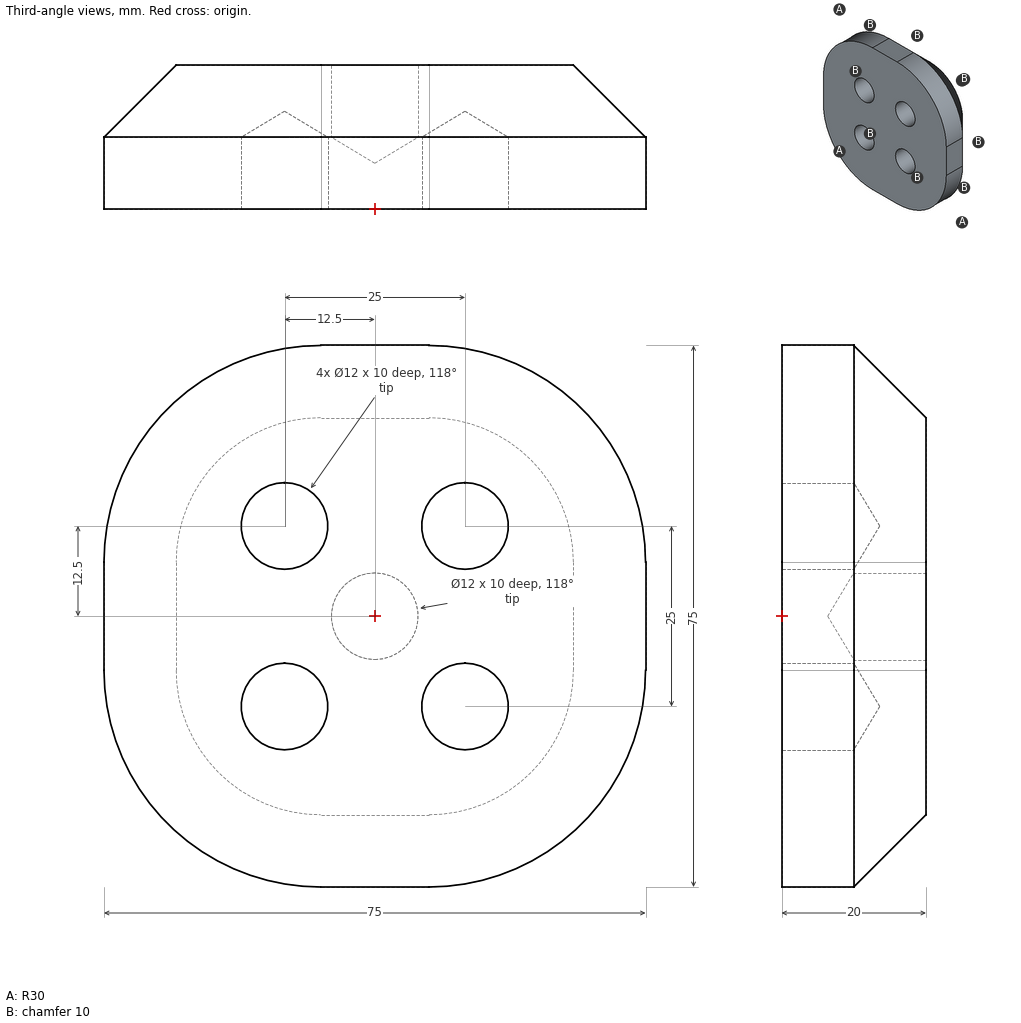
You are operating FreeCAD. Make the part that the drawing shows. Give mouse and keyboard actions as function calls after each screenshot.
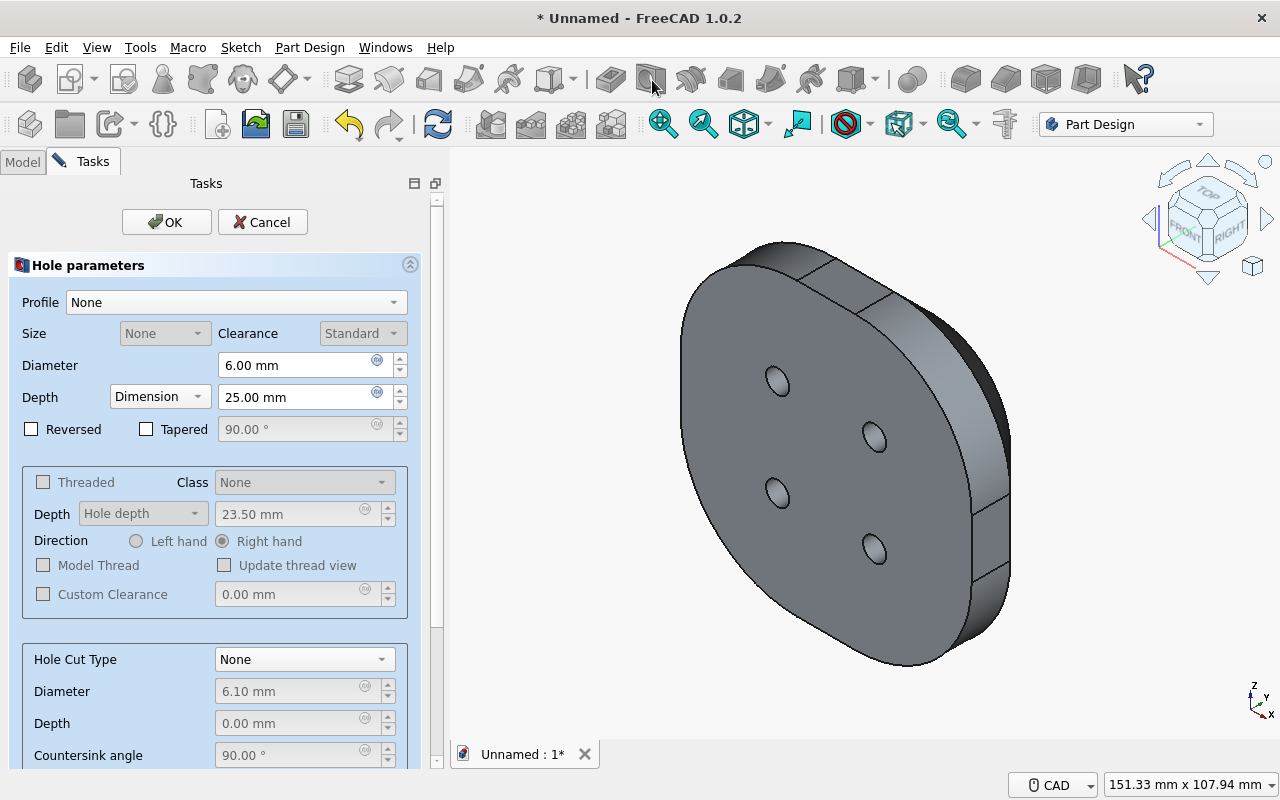
triple_click(305, 365)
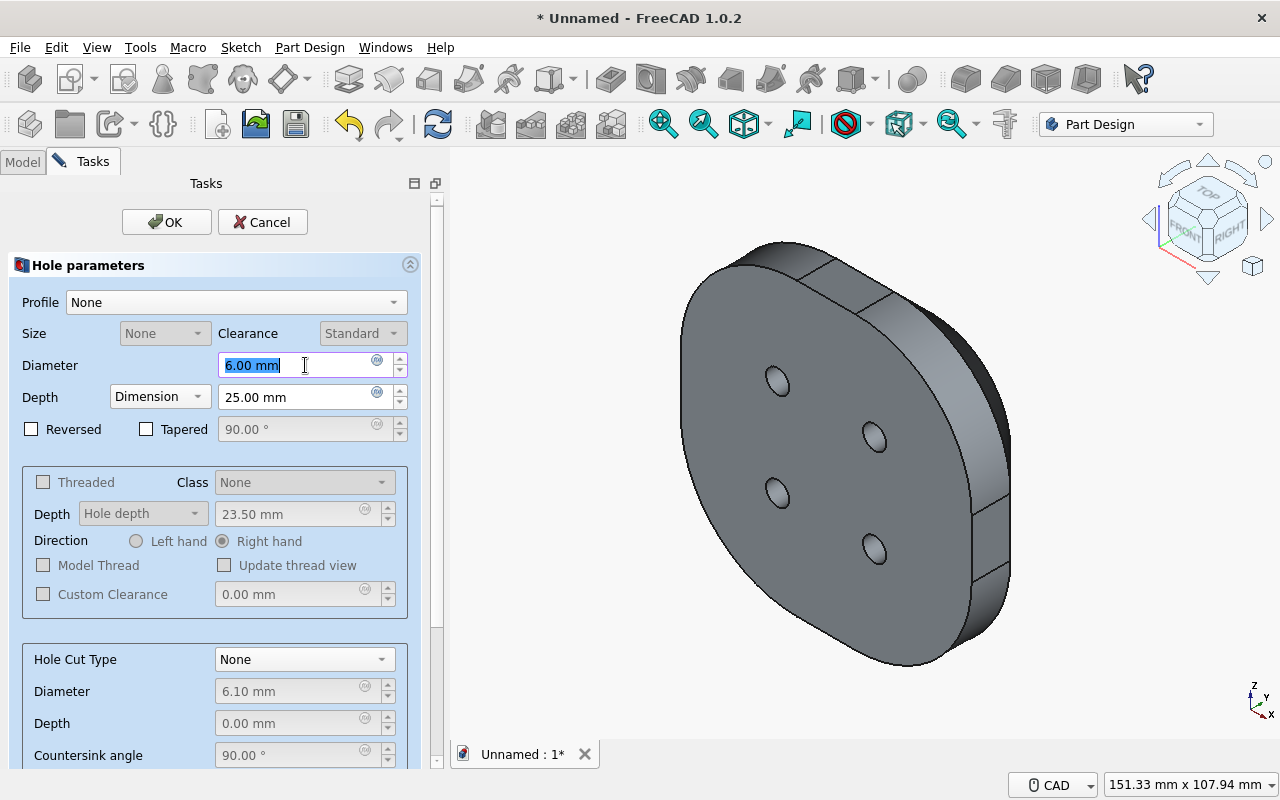
text(12)
key(Tab)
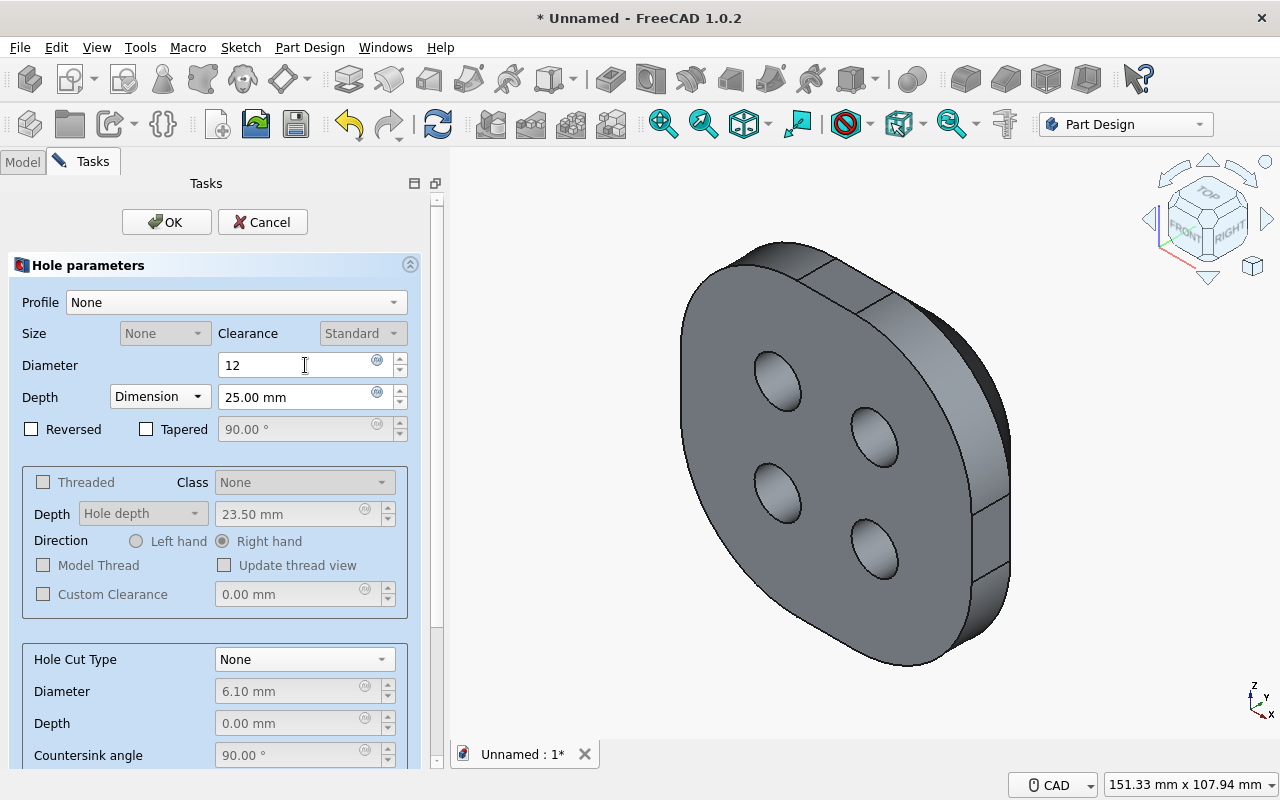
triple_click(305, 397)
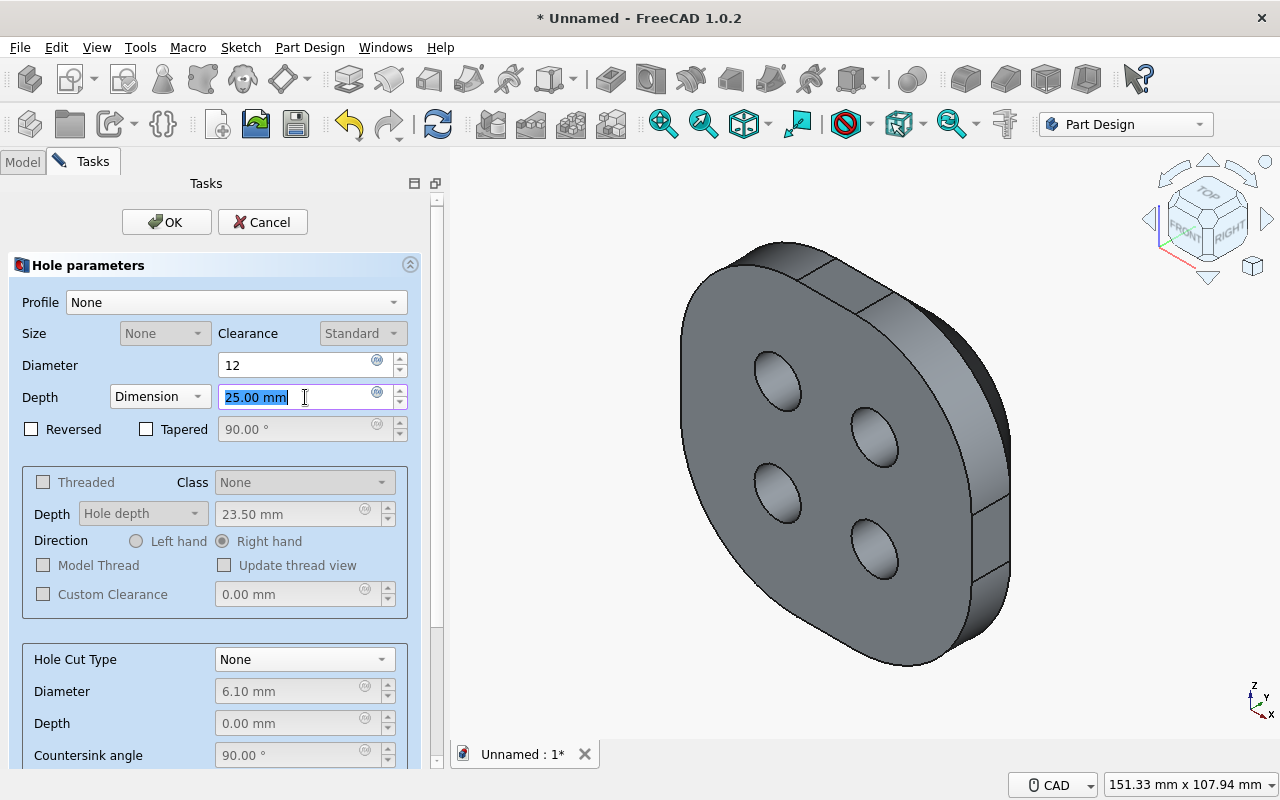
text(10)
key(Tab)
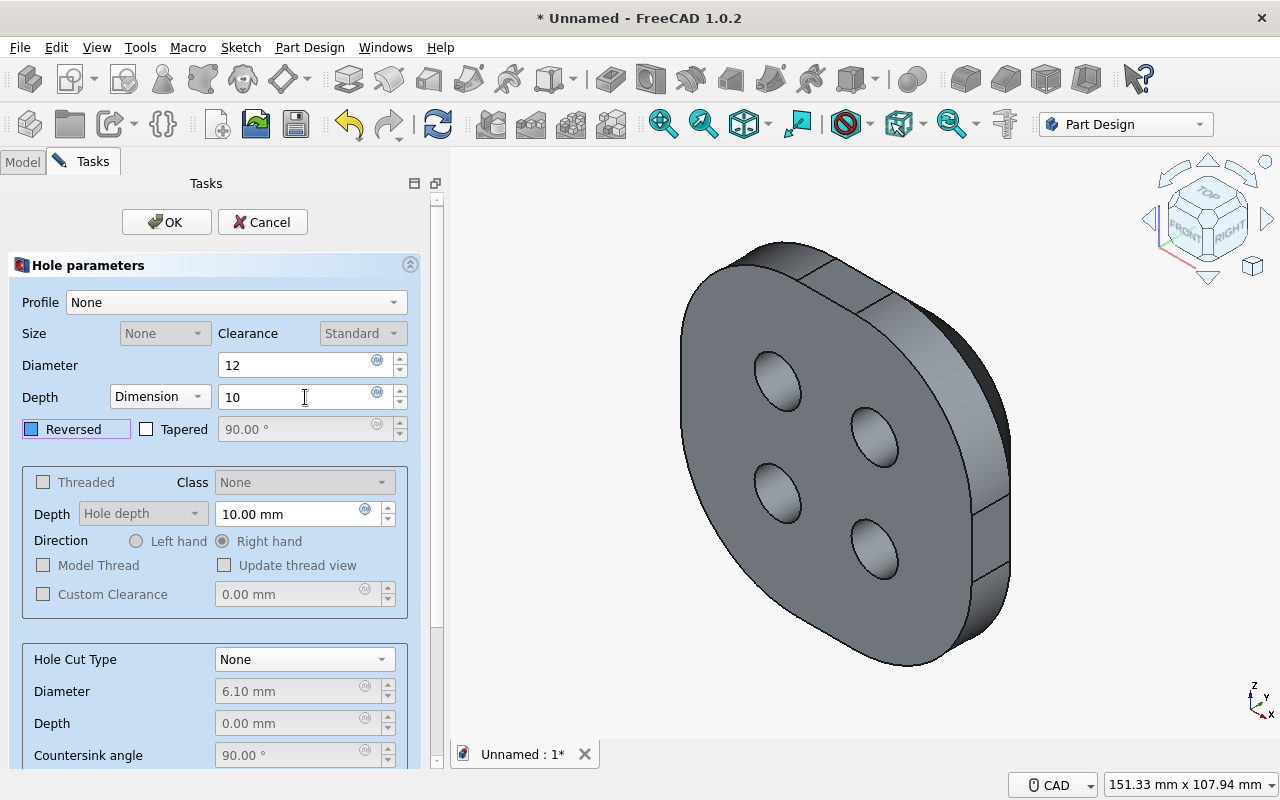
click(167, 222)